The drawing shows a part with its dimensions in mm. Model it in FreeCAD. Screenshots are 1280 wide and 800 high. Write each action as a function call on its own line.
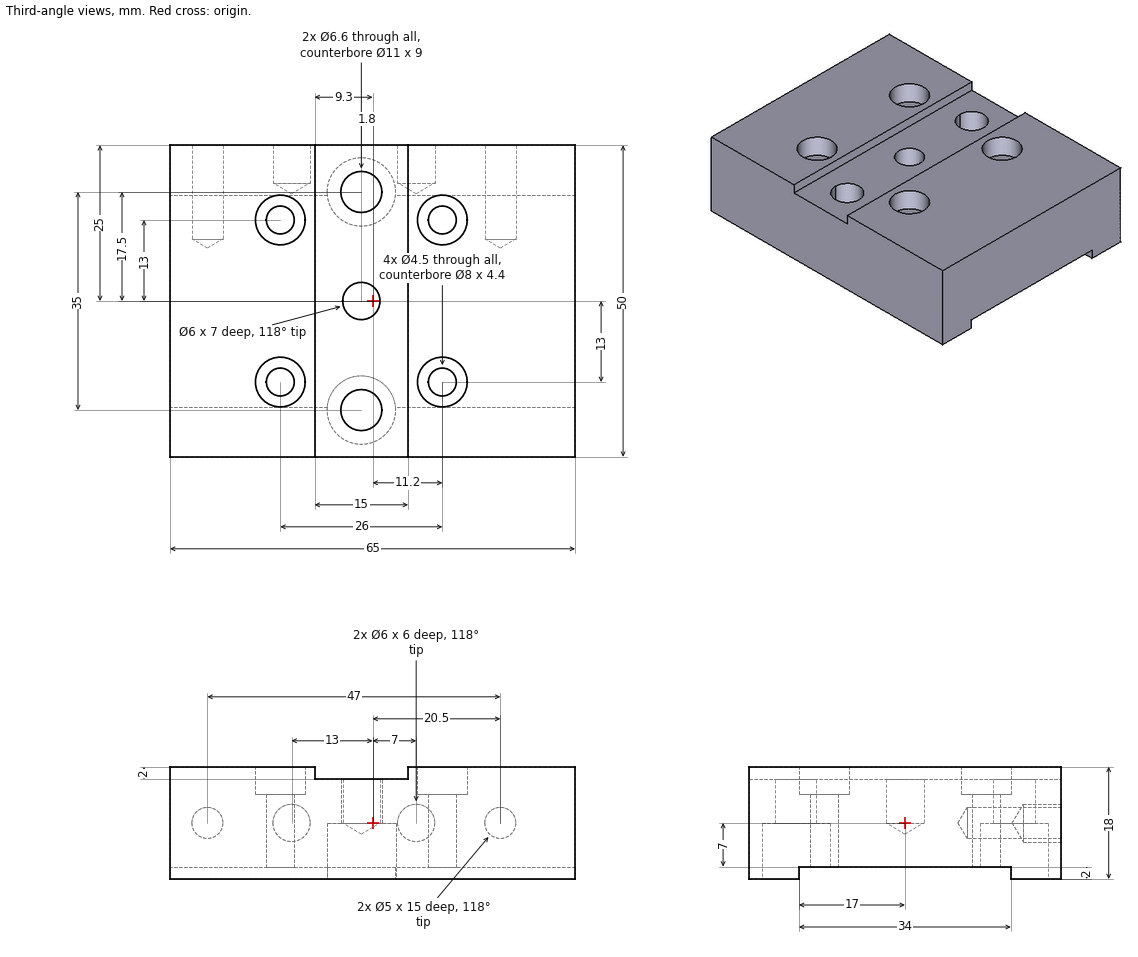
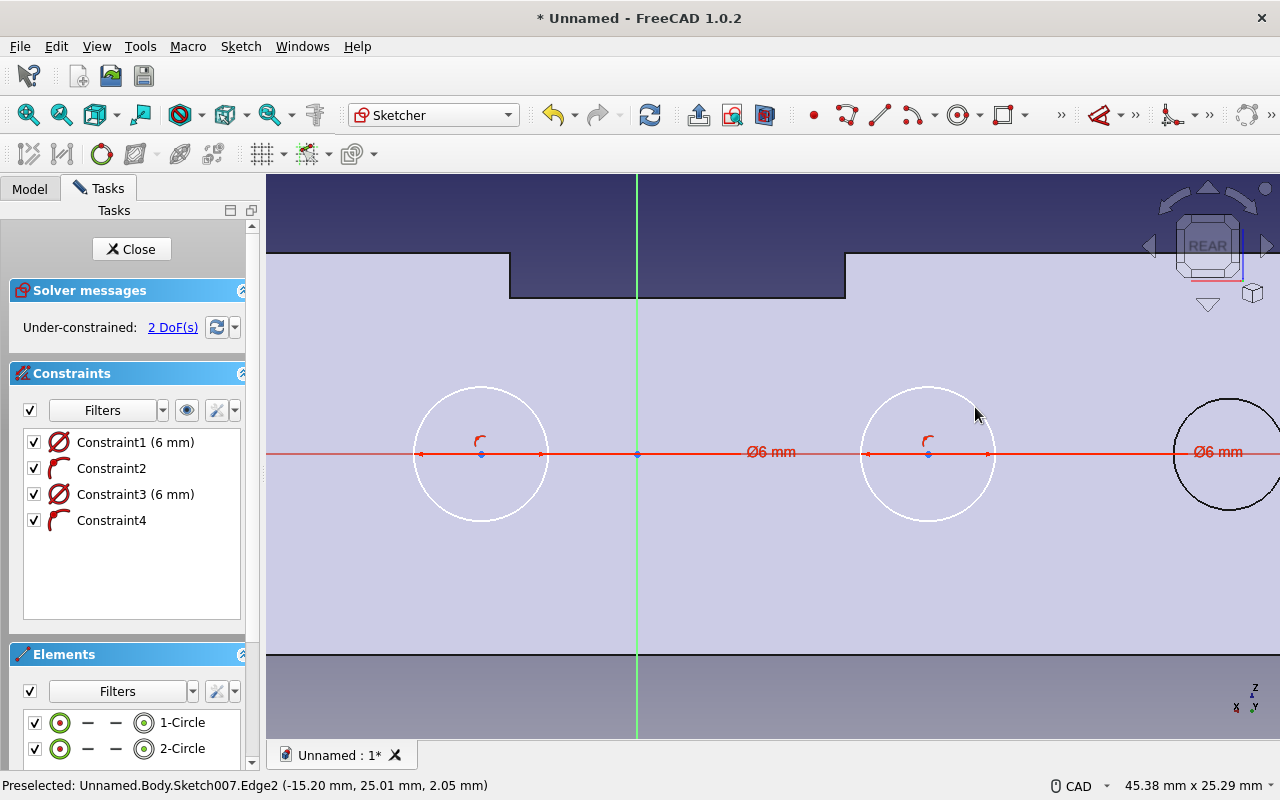
click(1098, 116)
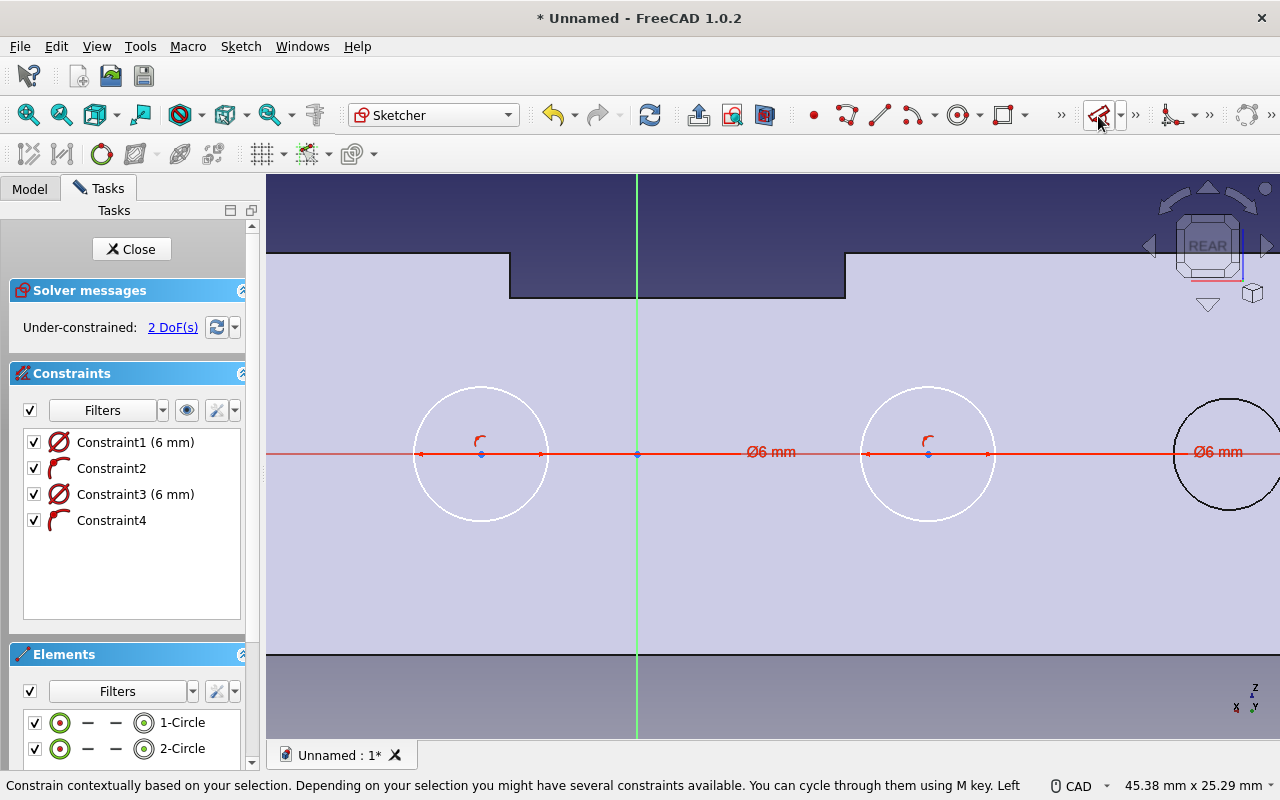
click(481, 454)
click(559, 488)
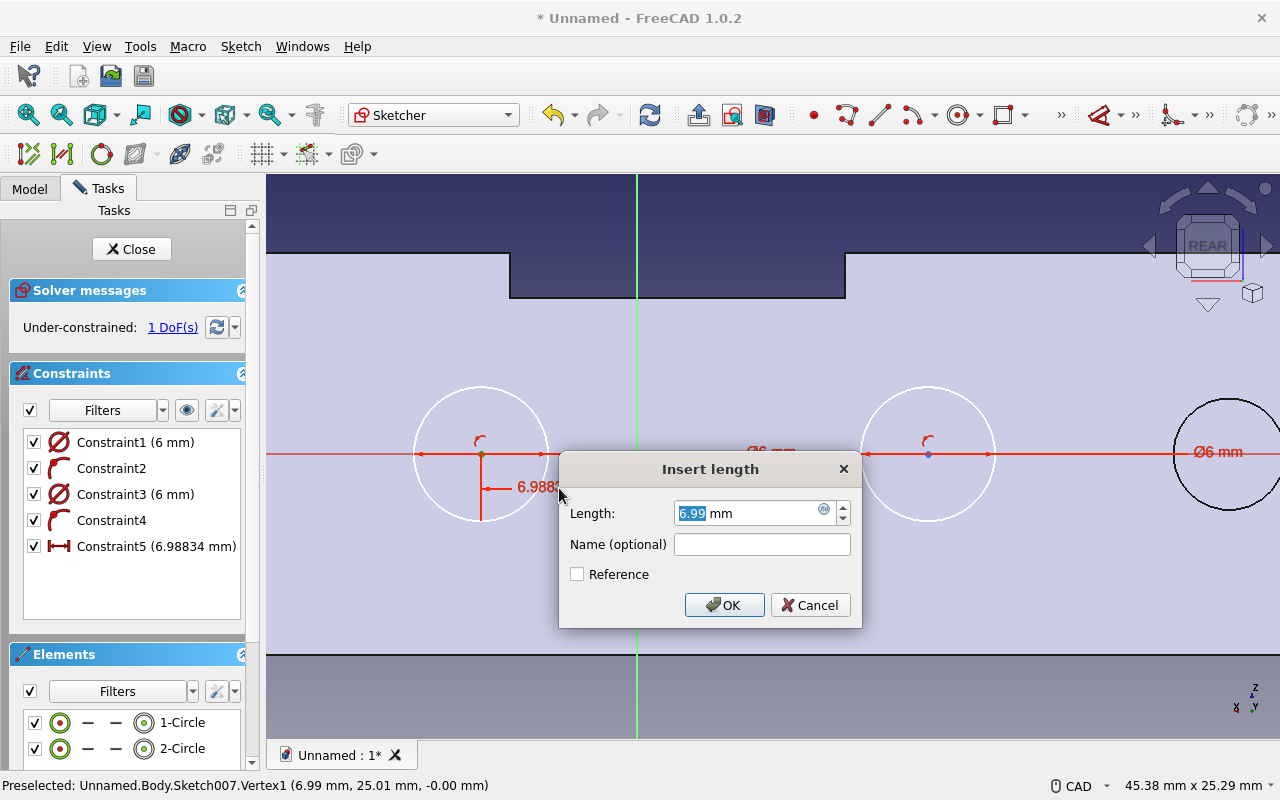
text(7)
key(Return)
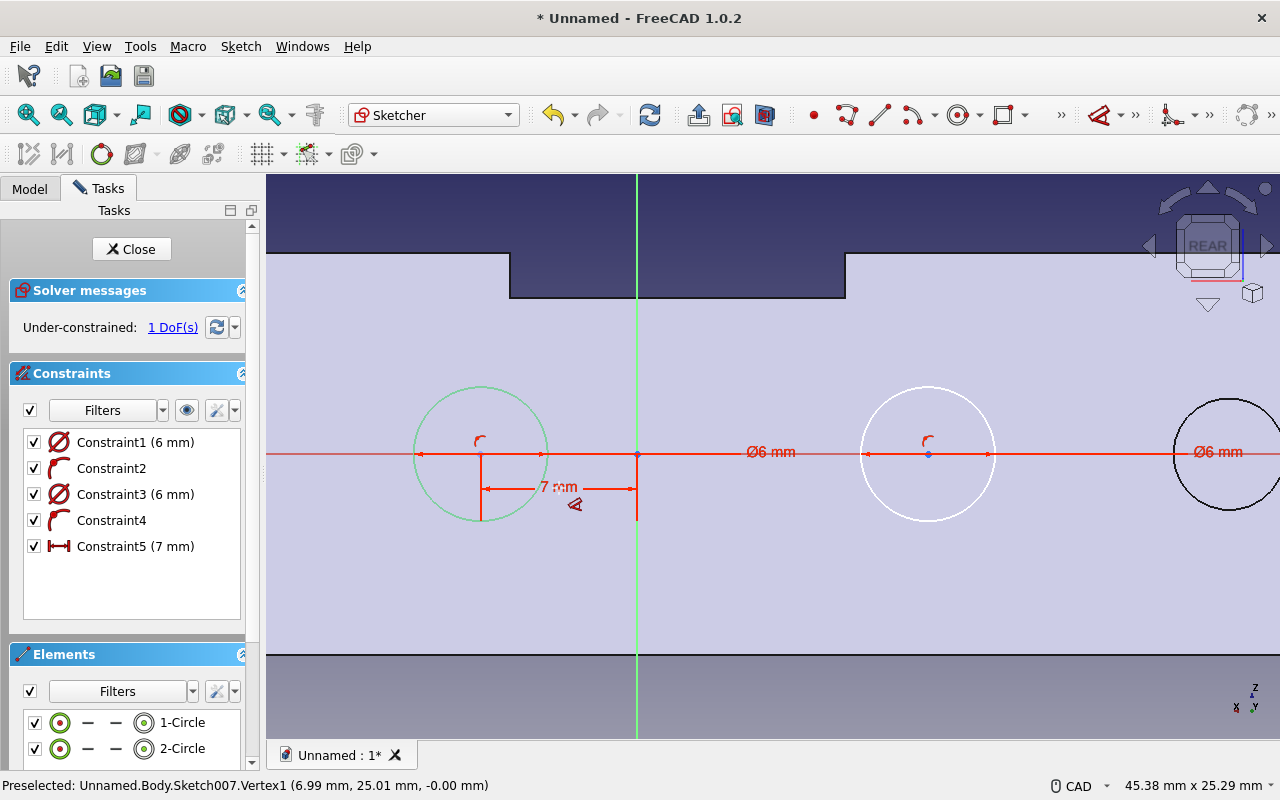
click(928, 454)
click(783, 488)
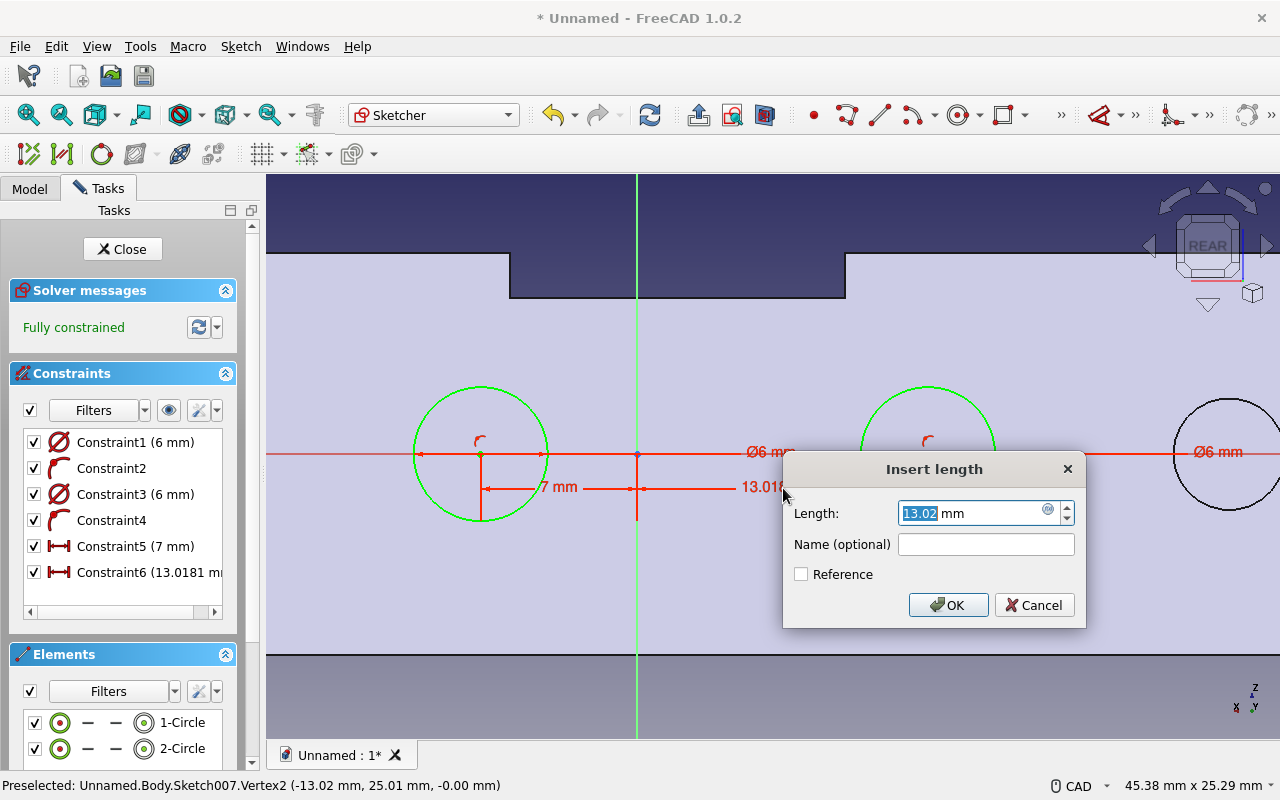
text(13)
key(Return)
key(Escape)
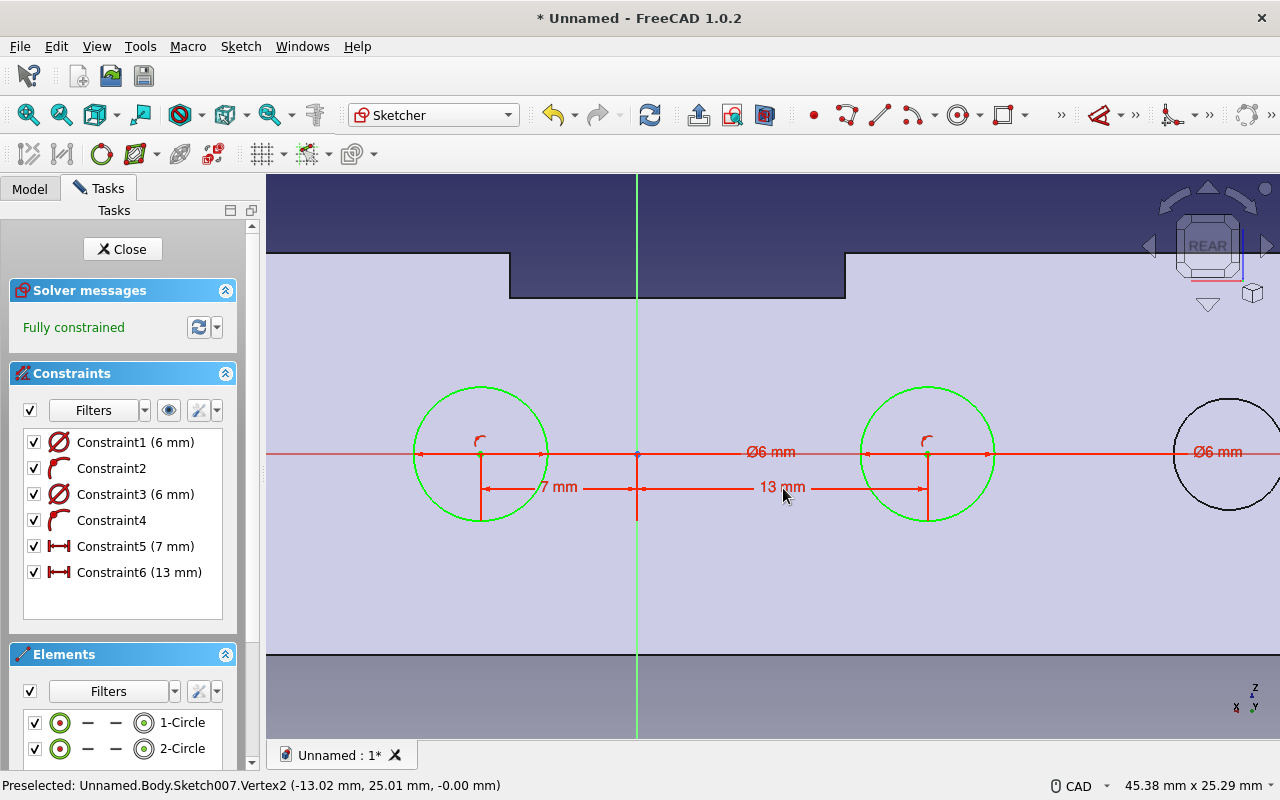
click(123, 249)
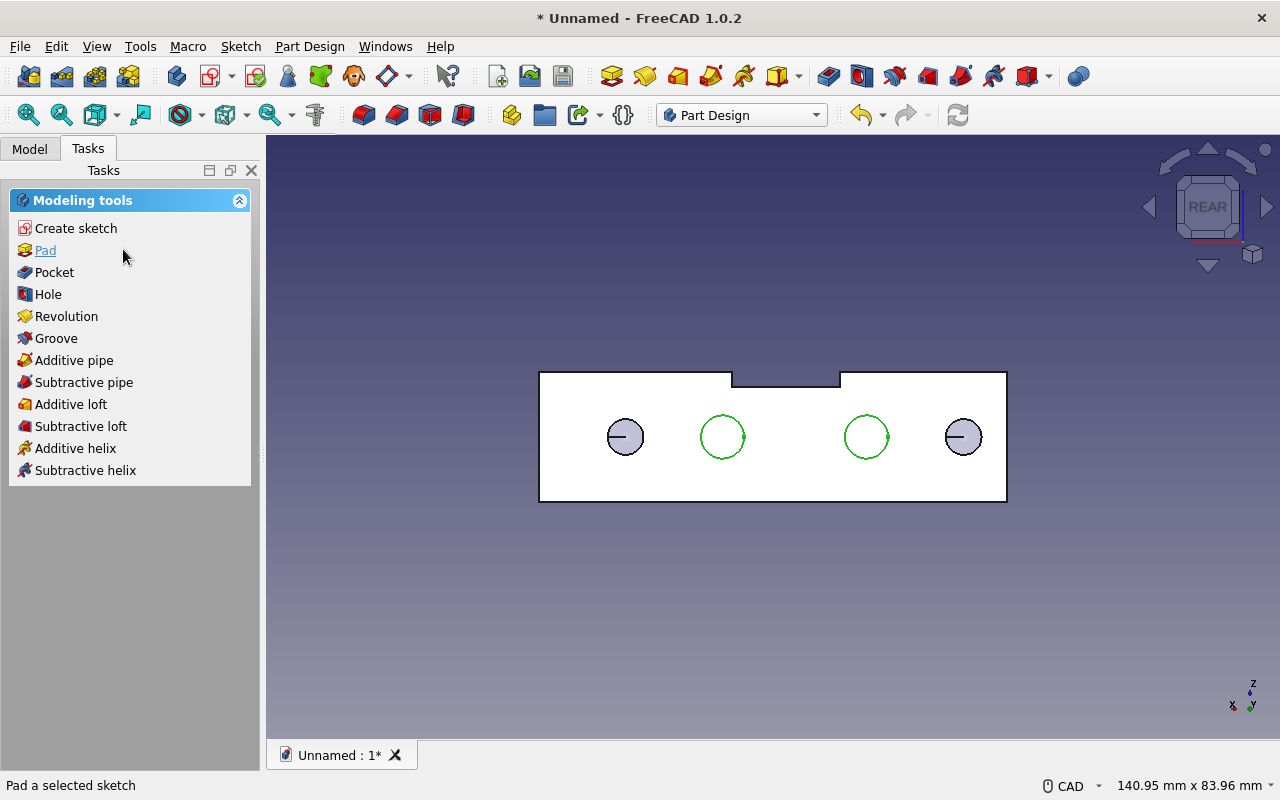
click(862, 76)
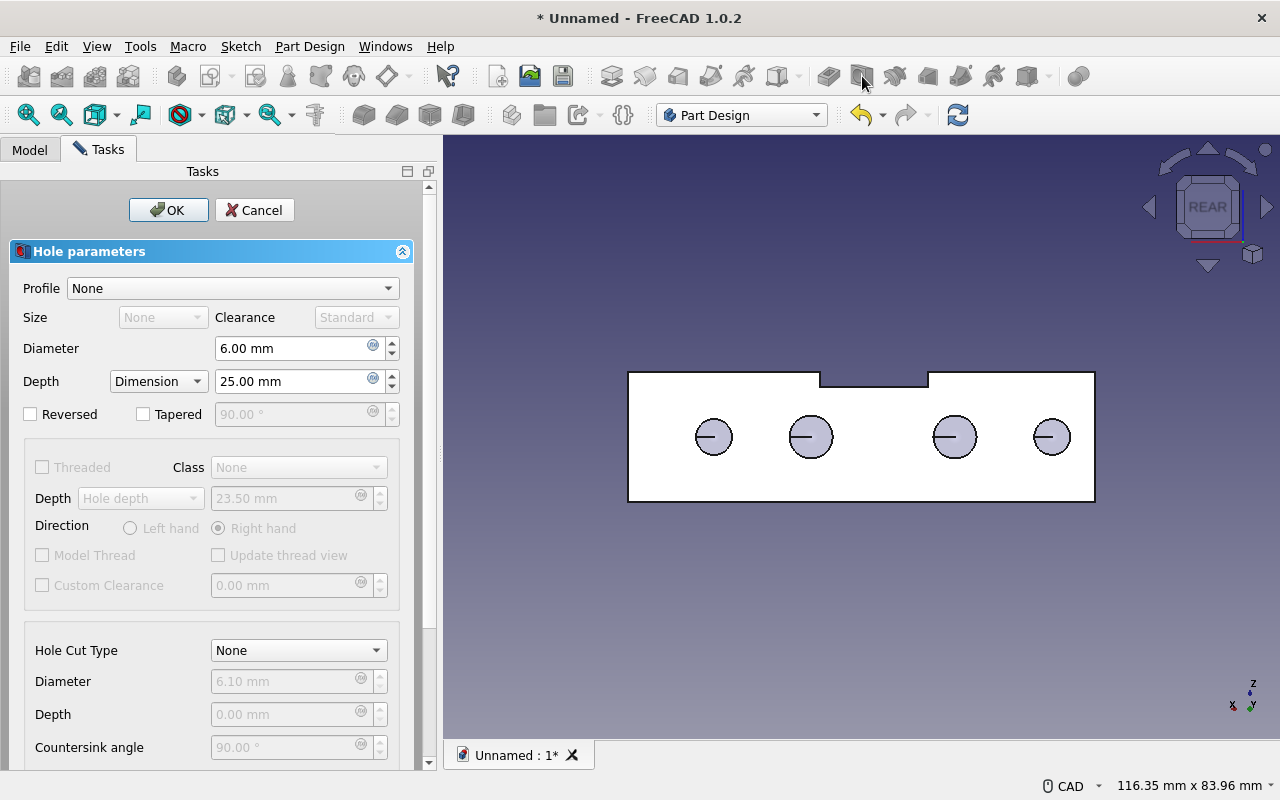
triple_click(300, 348)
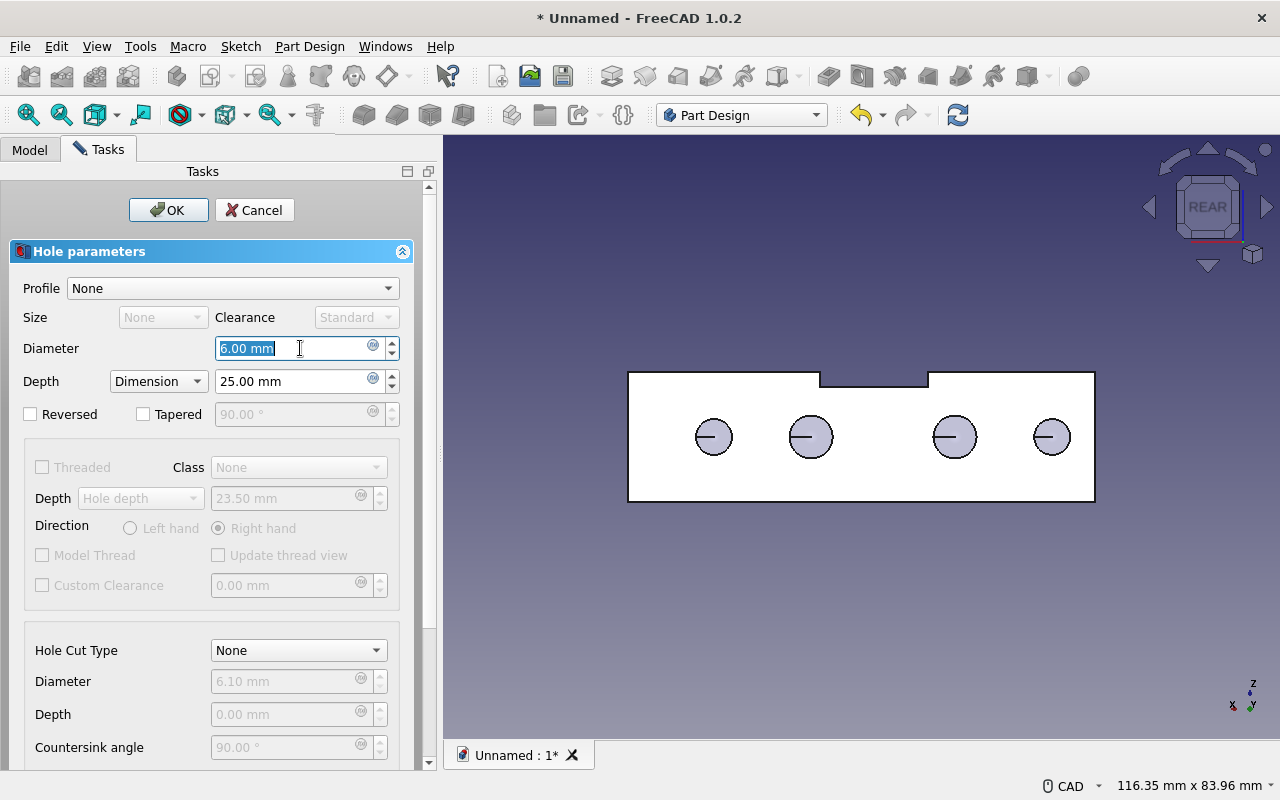
text(6)
key(Tab)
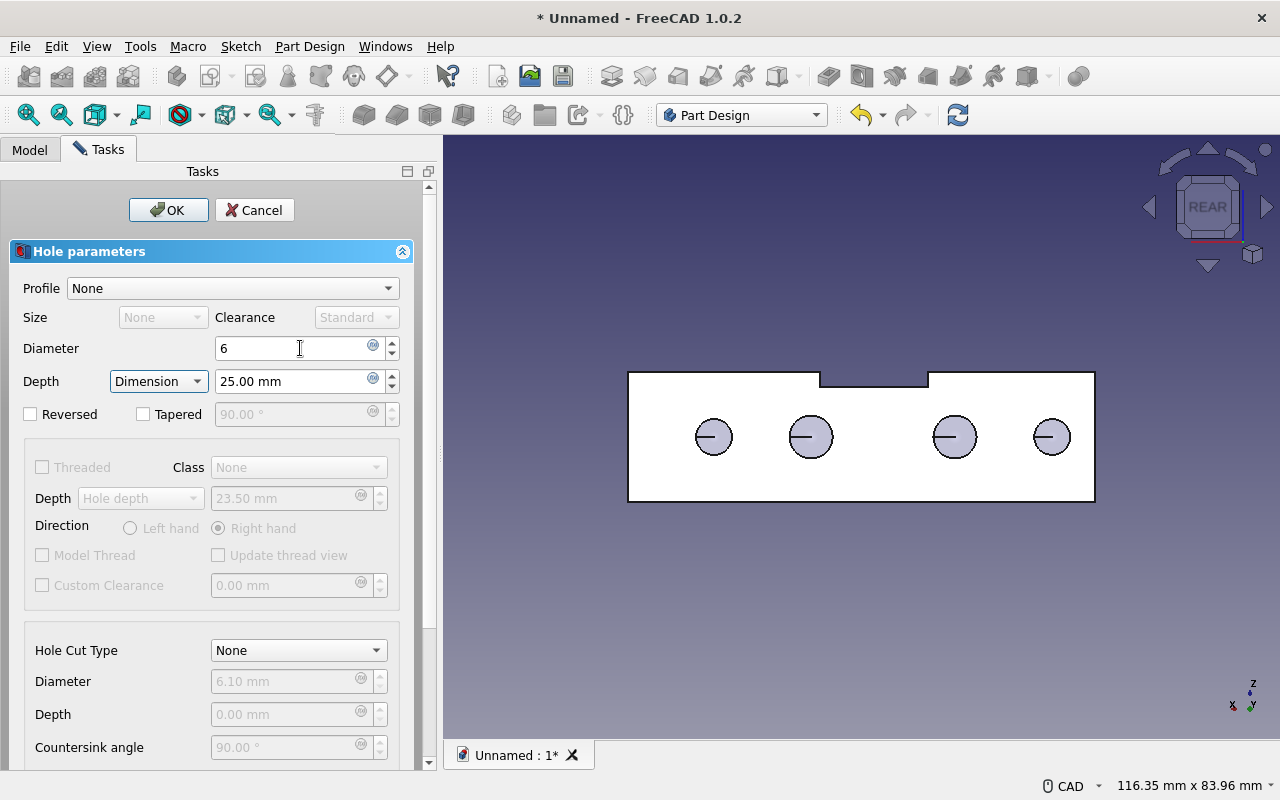
triple_click(300, 382)